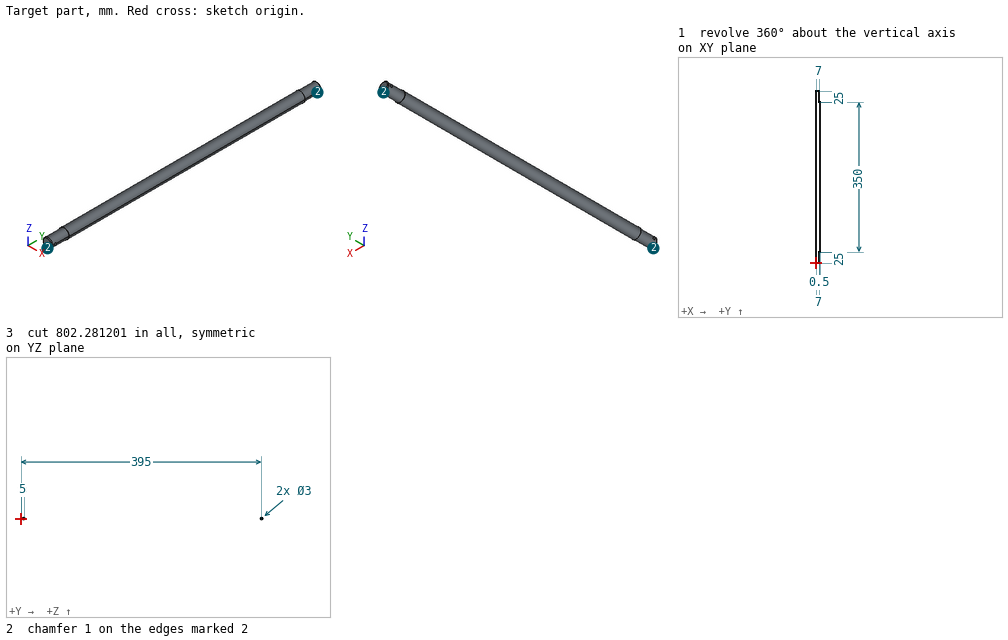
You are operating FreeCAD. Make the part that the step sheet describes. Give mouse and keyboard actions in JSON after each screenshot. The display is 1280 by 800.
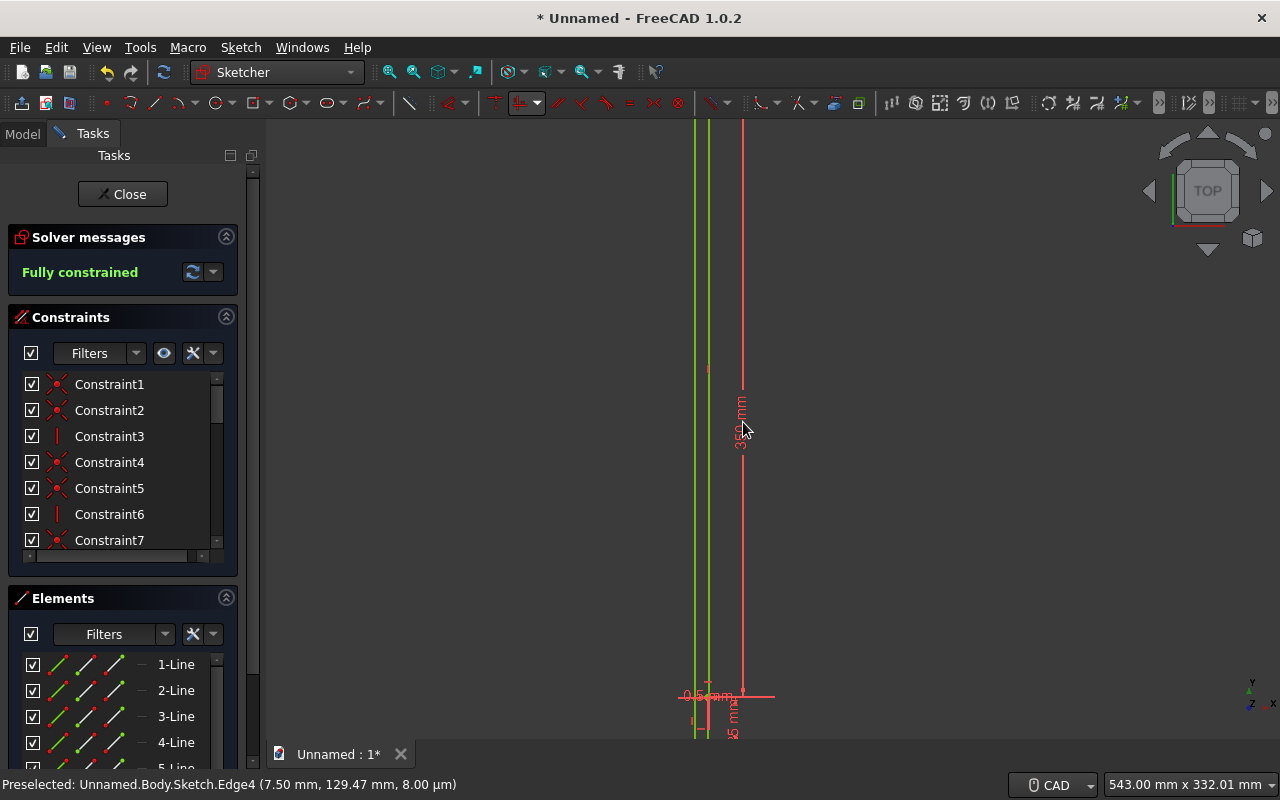
{"action": "left_click", "coordinate": [123, 194]}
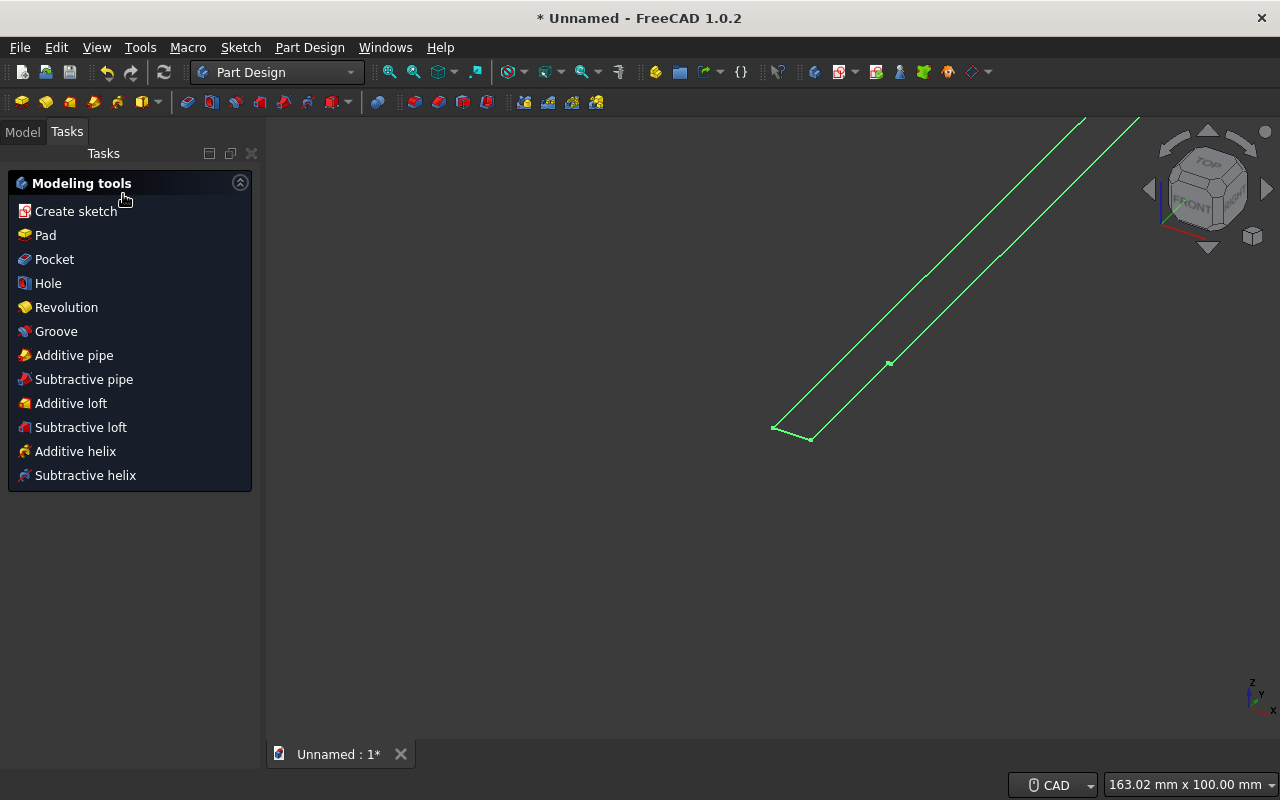
{"action": "left_click", "coordinate": [46, 102]}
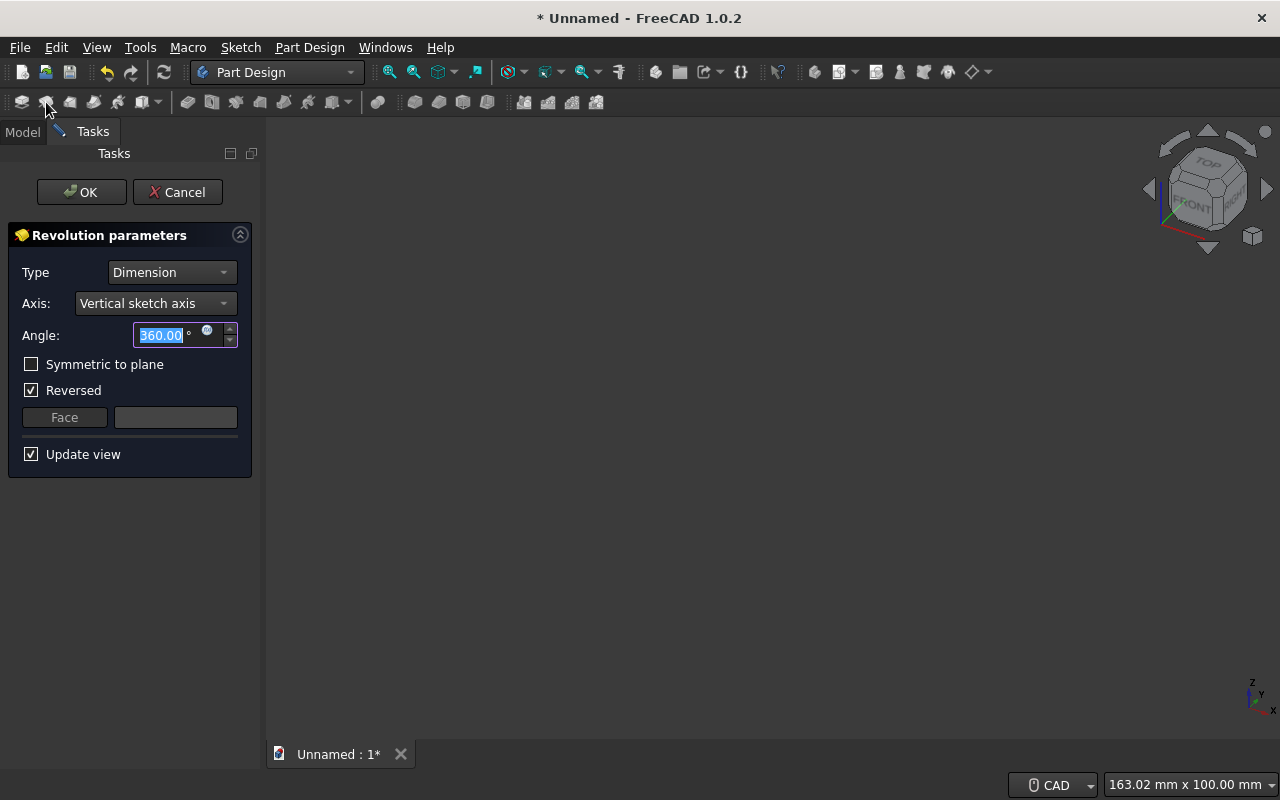
{"action": "left_click", "coordinate": [82, 192]}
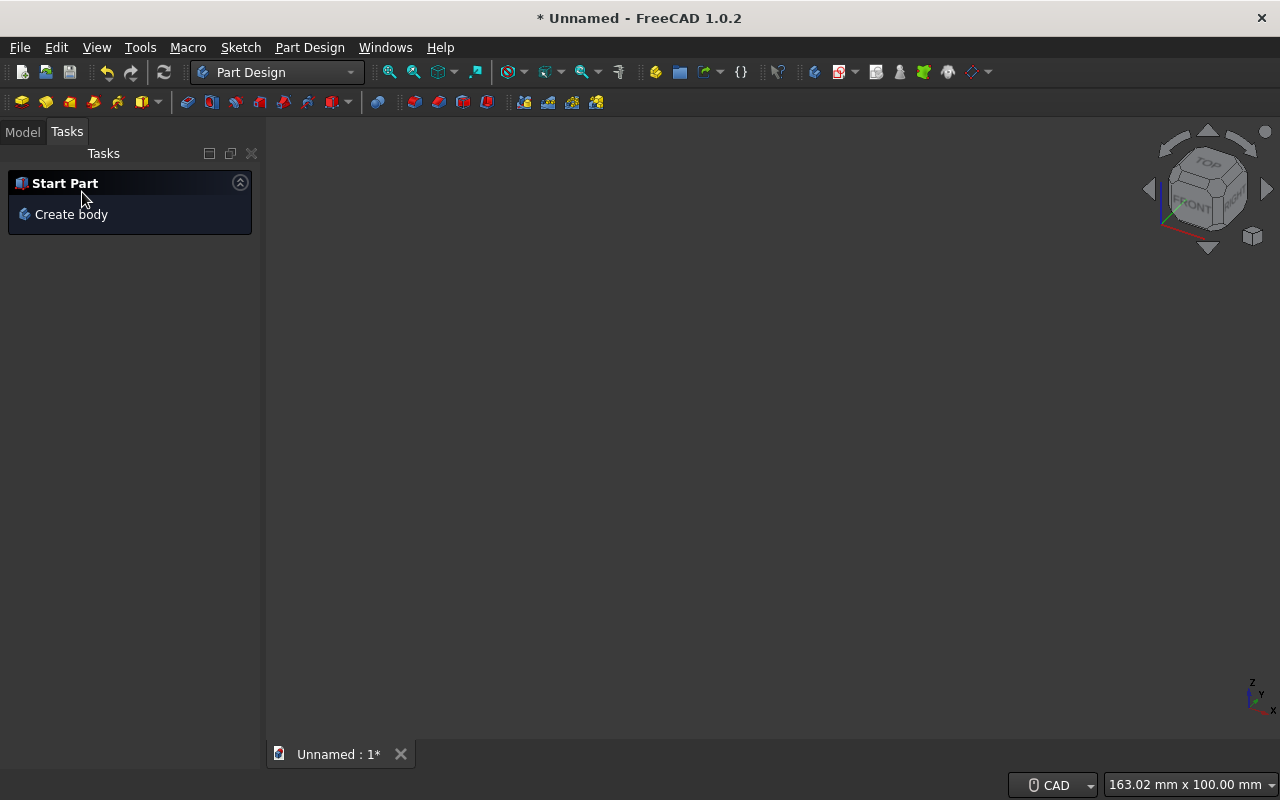
{"action": "left_click", "coordinate": [390, 72]}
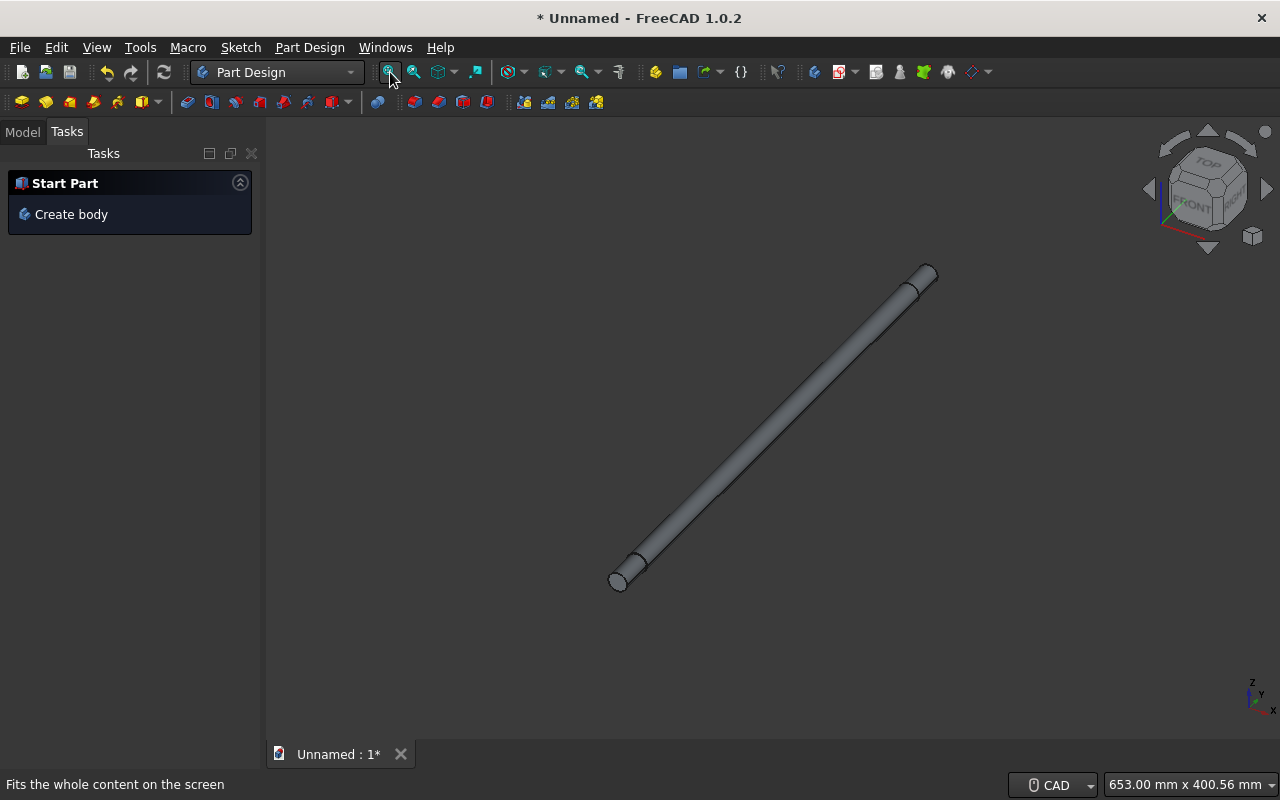
{"action": "left_click", "coordinate": [925, 263]}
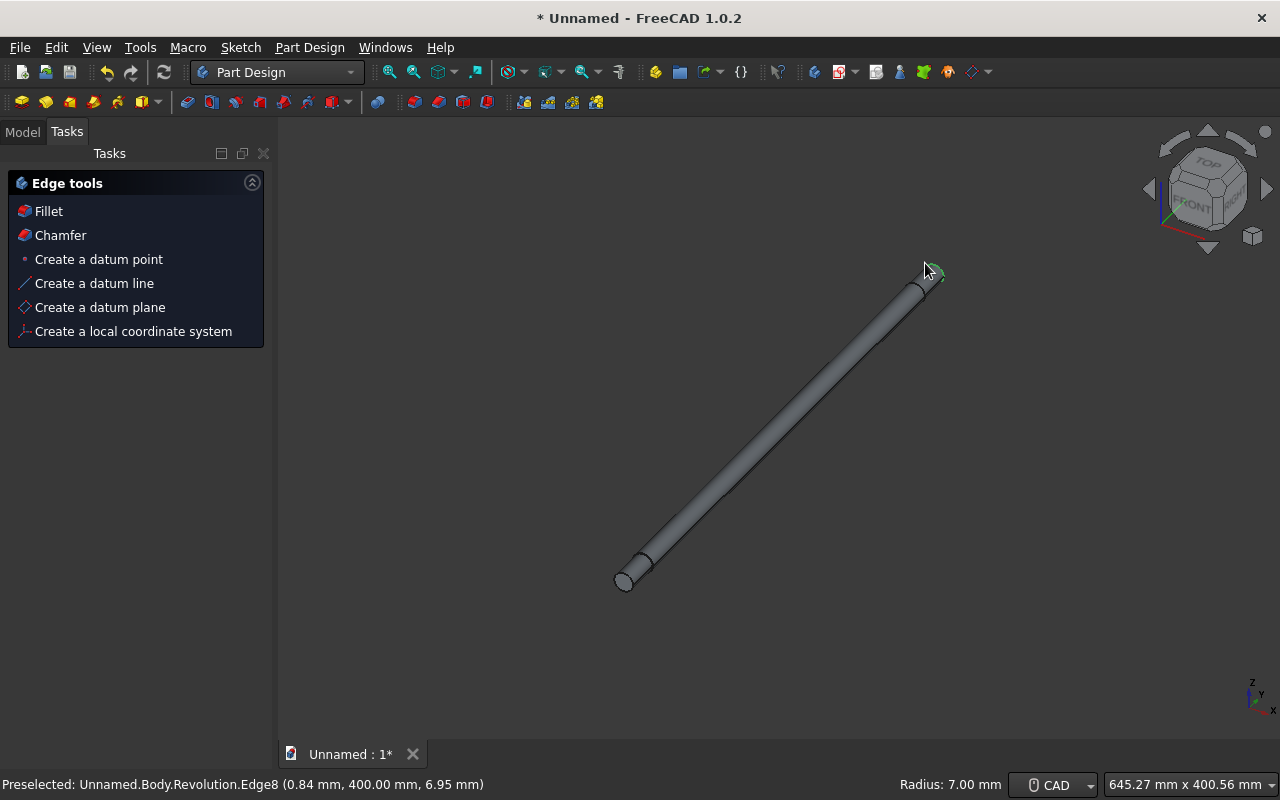
{"action": "left_click", "coordinate": [614, 578], "text": "ctrl"}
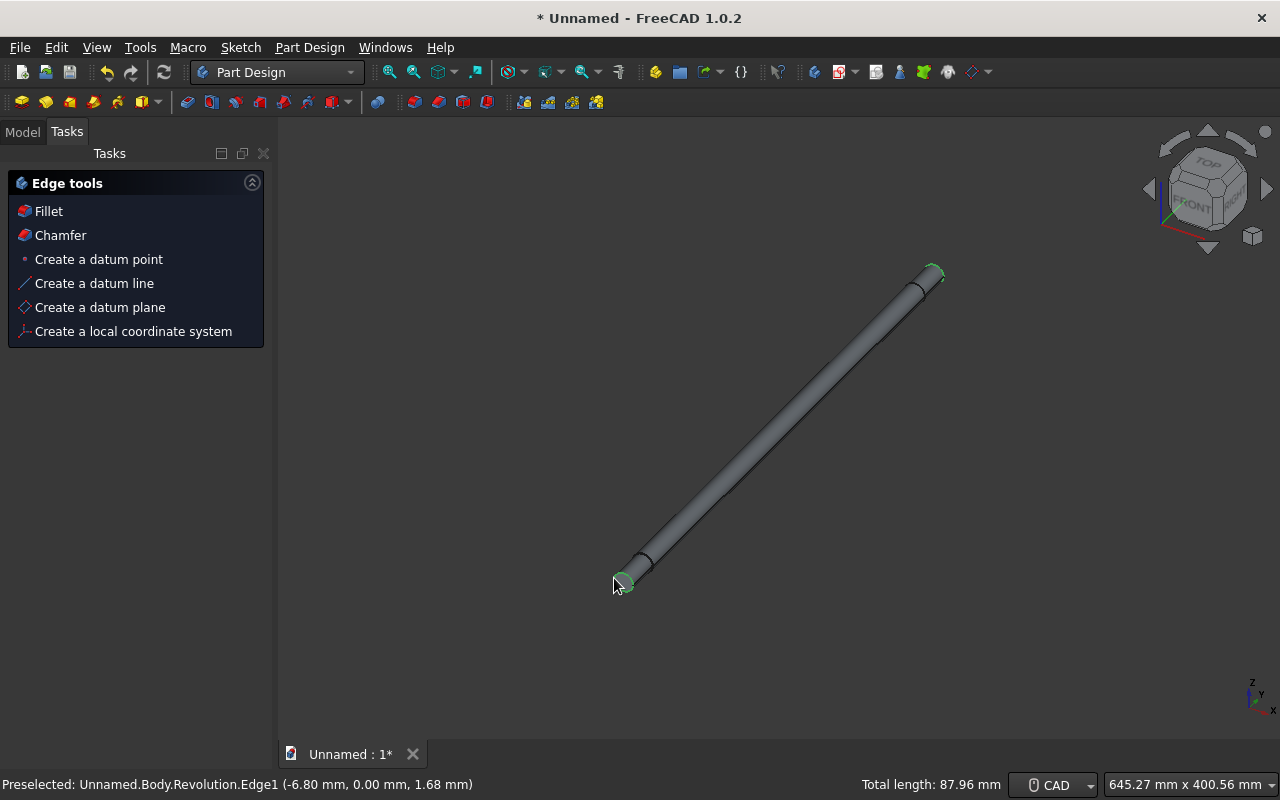
{"action": "left_click", "coordinate": [440, 102]}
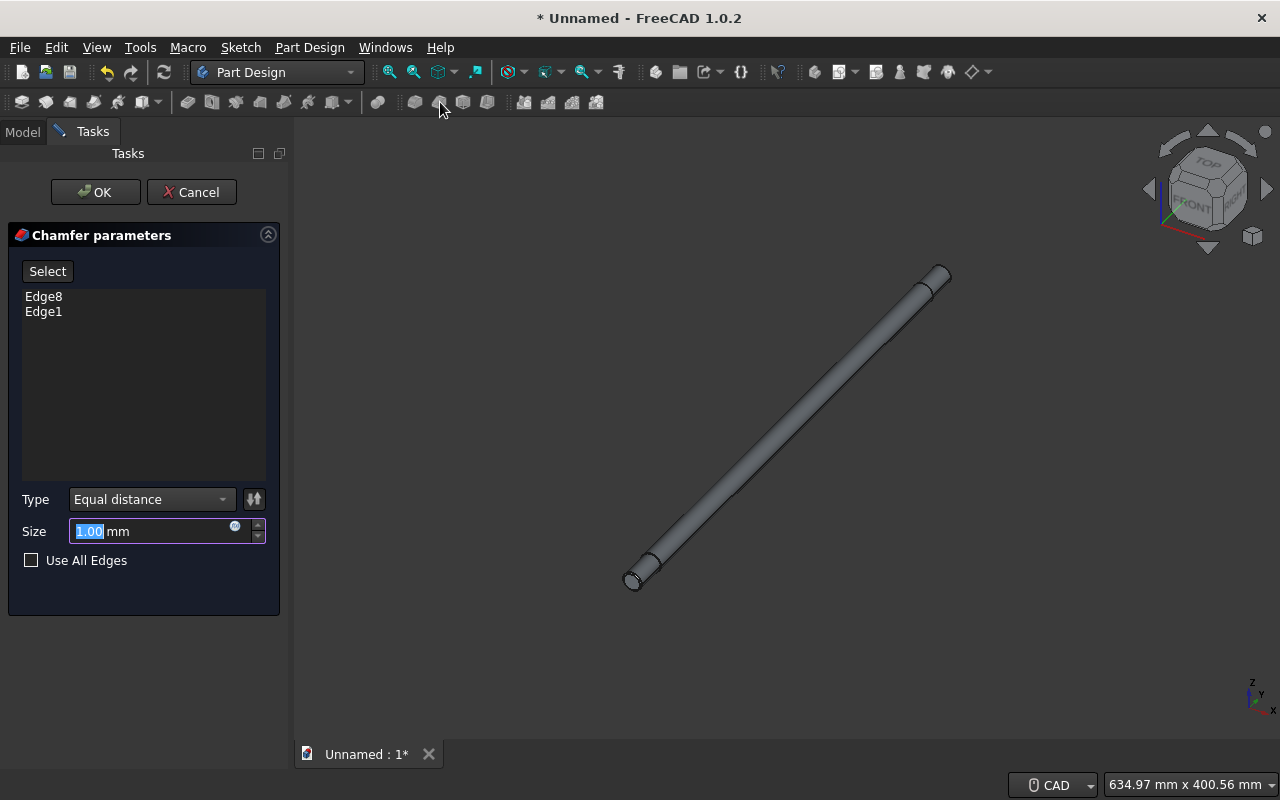
{"action": "type", "text": "1"}
{"action": "key", "text": "Tab"}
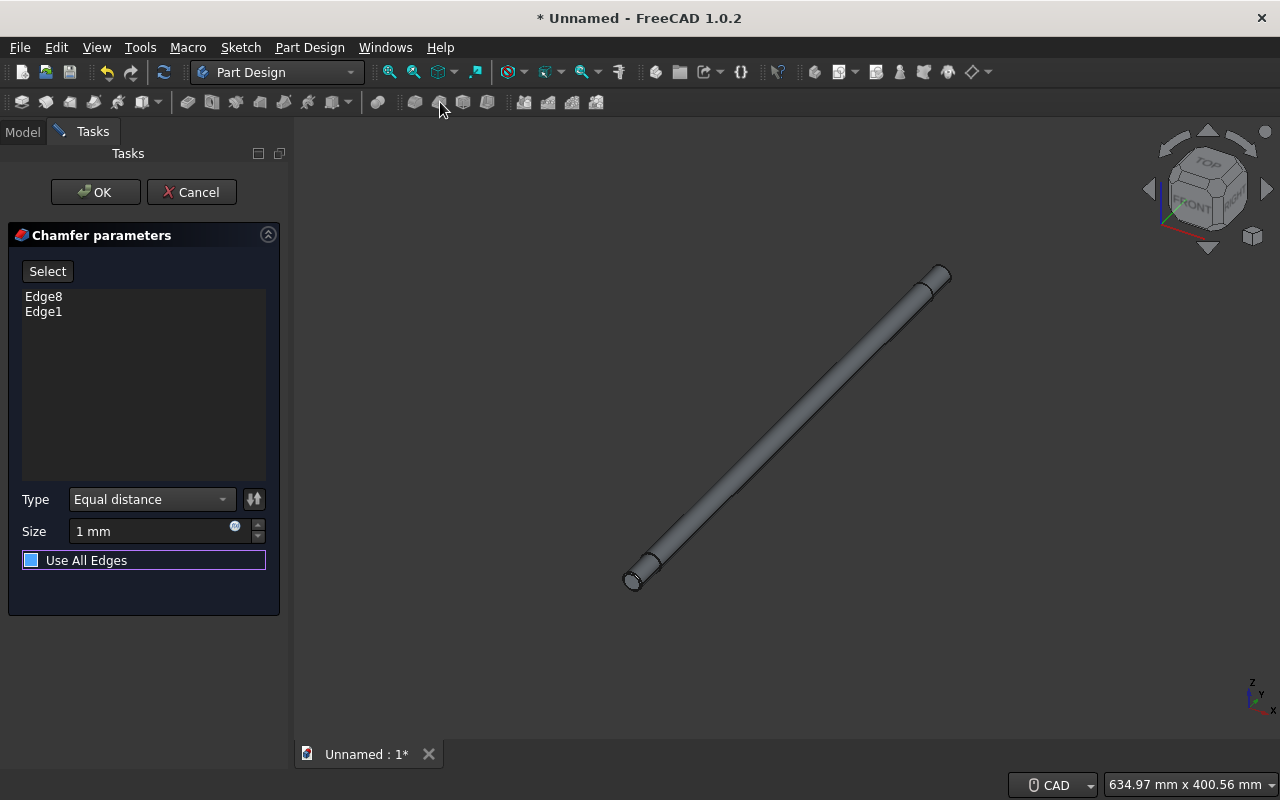
{"action": "left_click", "coordinate": [96, 192]}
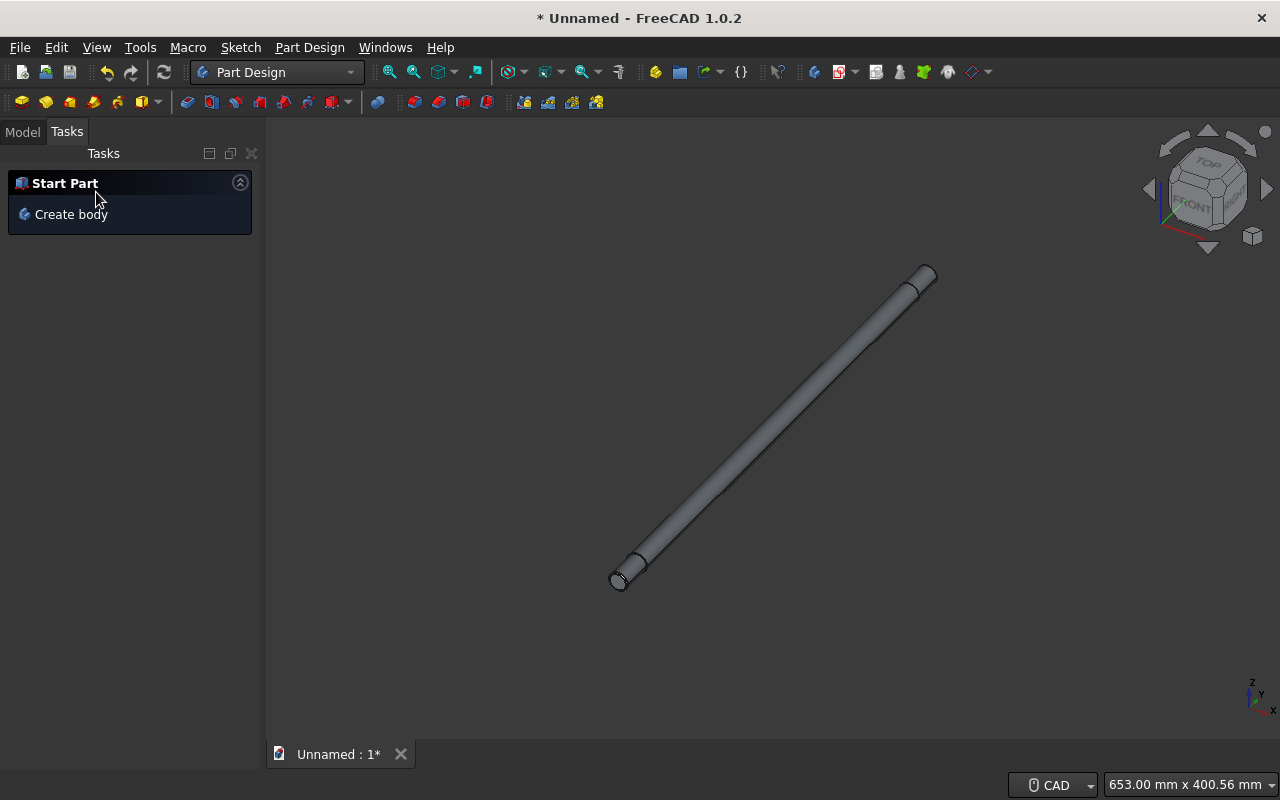
{"action": "left_click", "coordinate": [840, 72]}